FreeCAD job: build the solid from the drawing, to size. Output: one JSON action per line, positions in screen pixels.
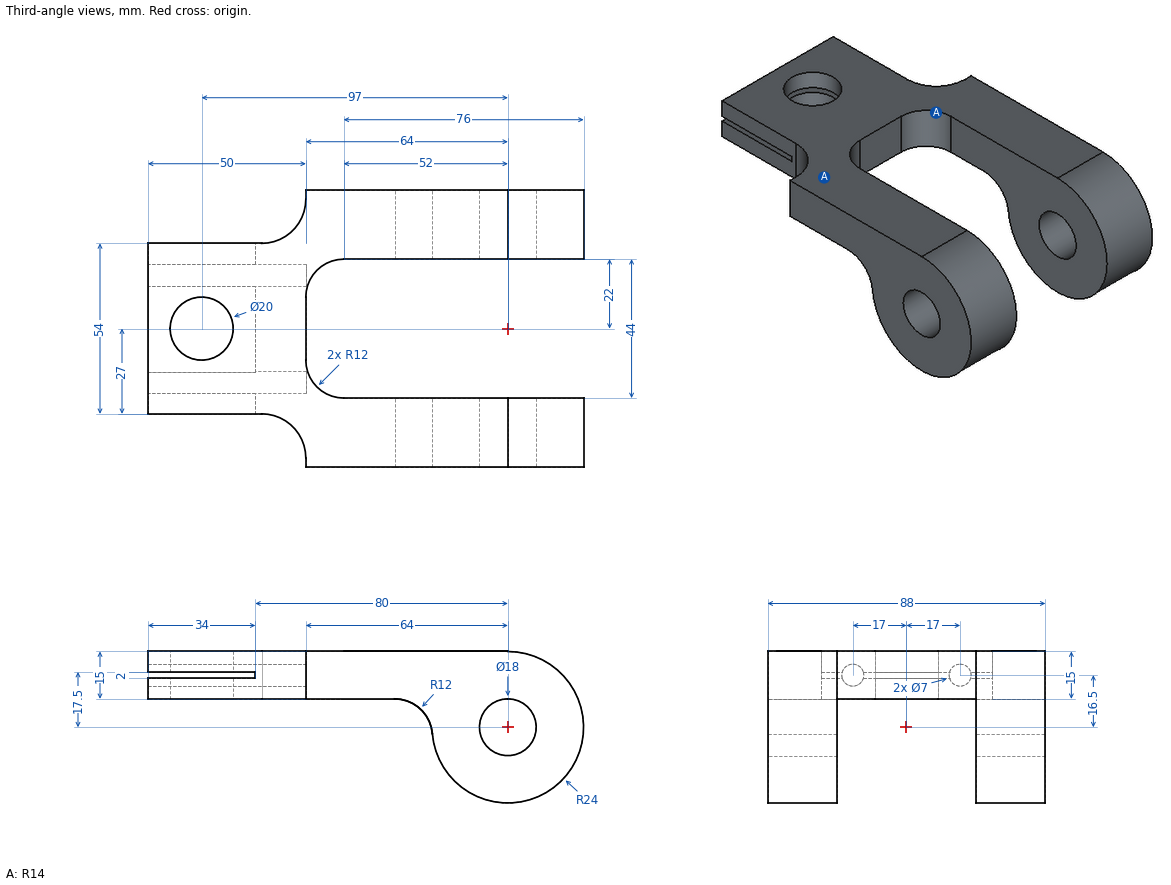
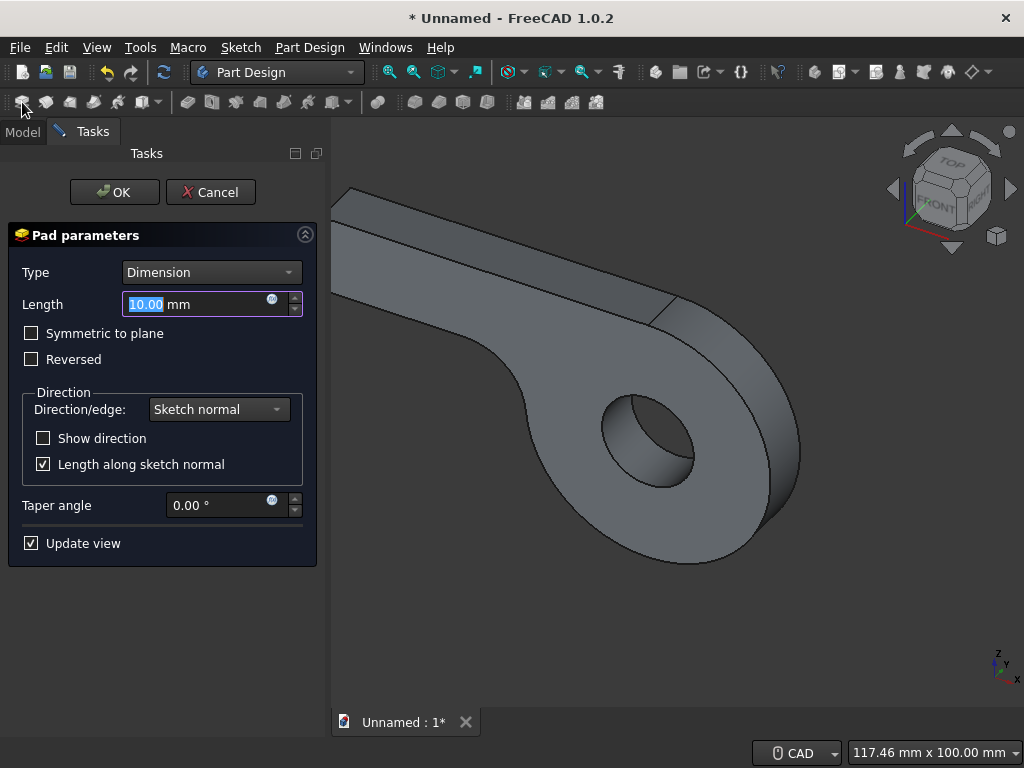
{"action": "type", "text": "88"}
{"action": "key", "text": "Tab"}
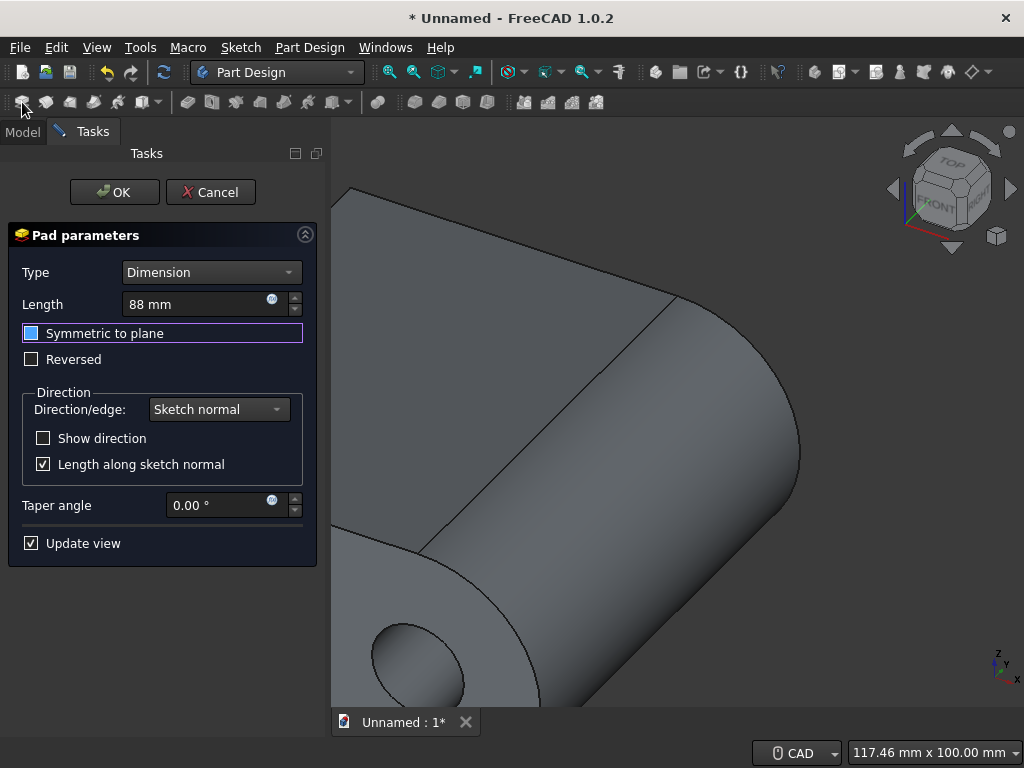
{"action": "left_click", "coordinate": [30, 333]}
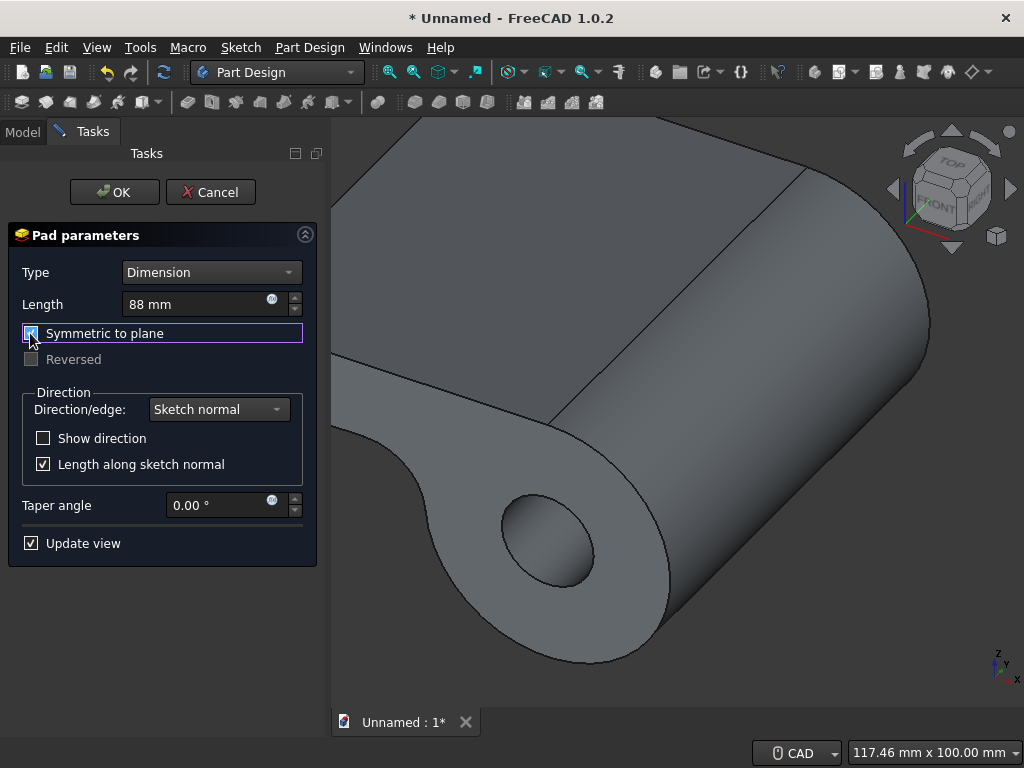
{"action": "left_click", "coordinate": [115, 192]}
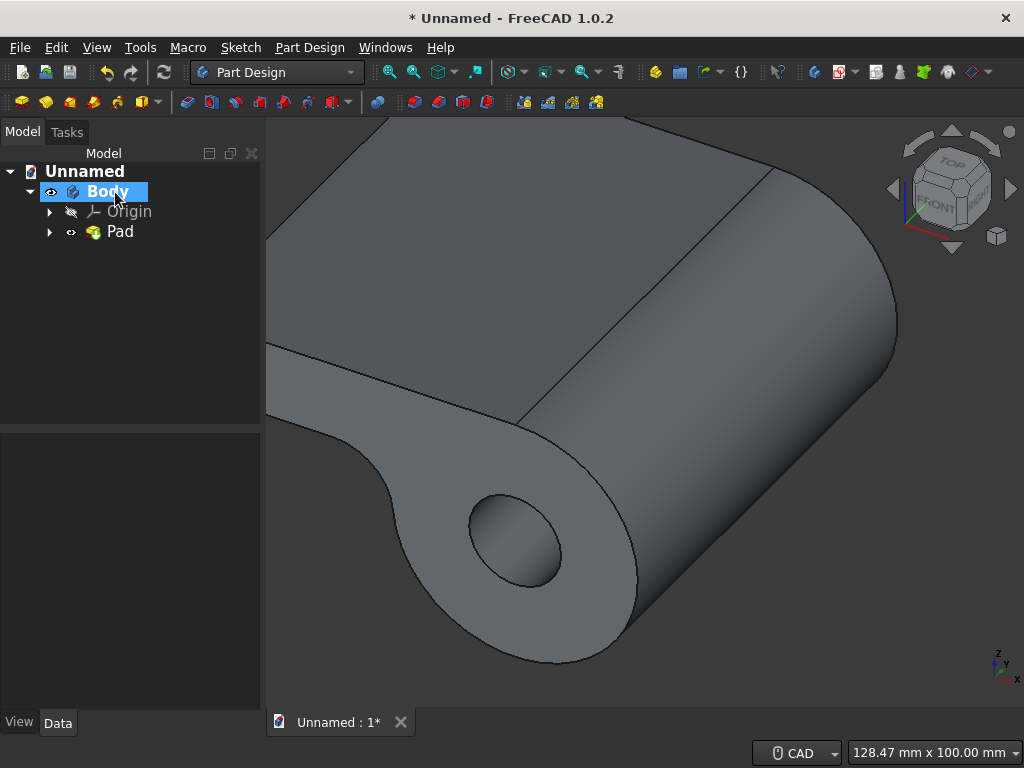
{"action": "left_click", "coordinate": [390, 72]}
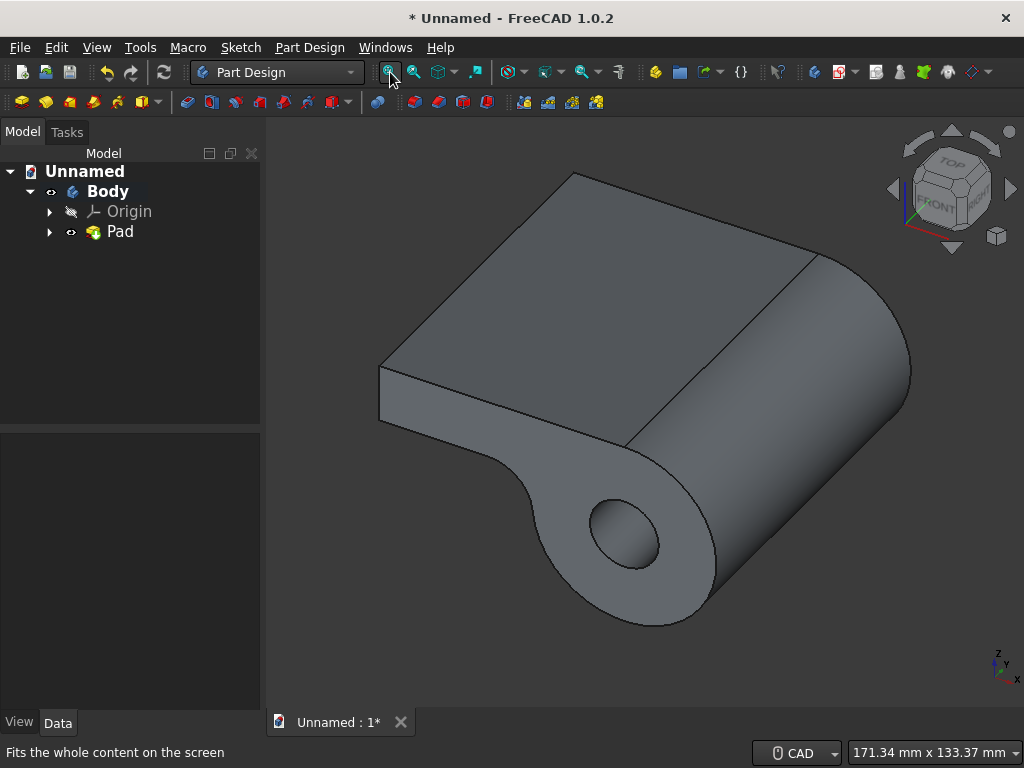
{"action": "key", "text": "5"}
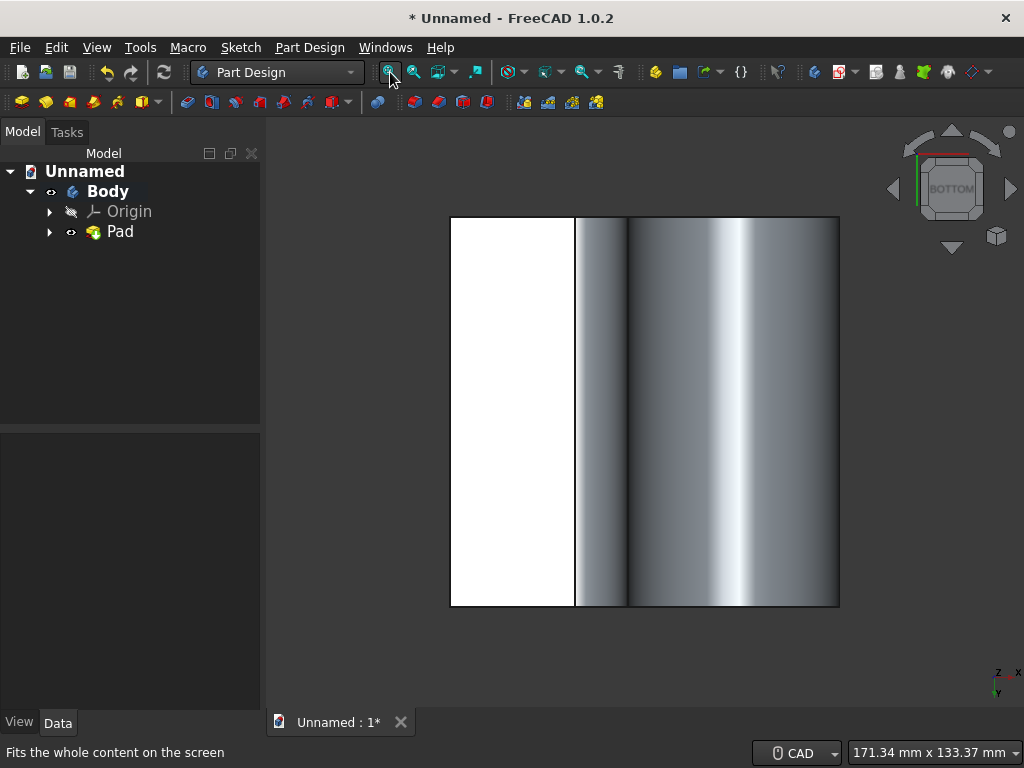
{"action": "left_click", "coordinate": [513, 522]}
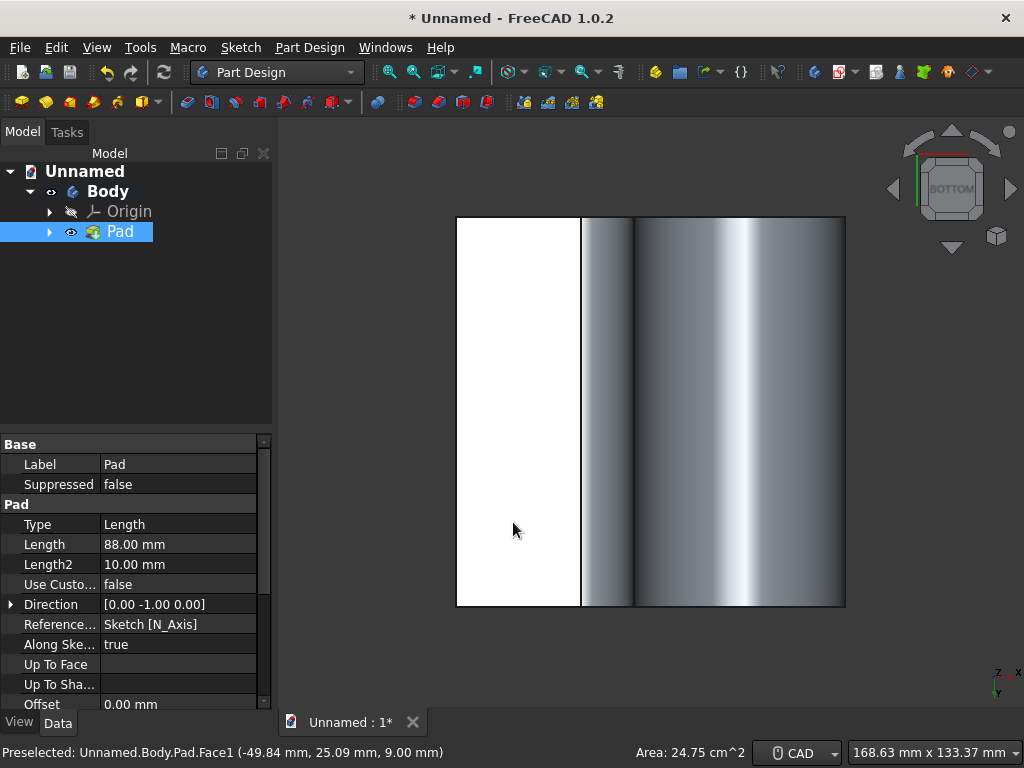
{"action": "left_click", "coordinate": [840, 72]}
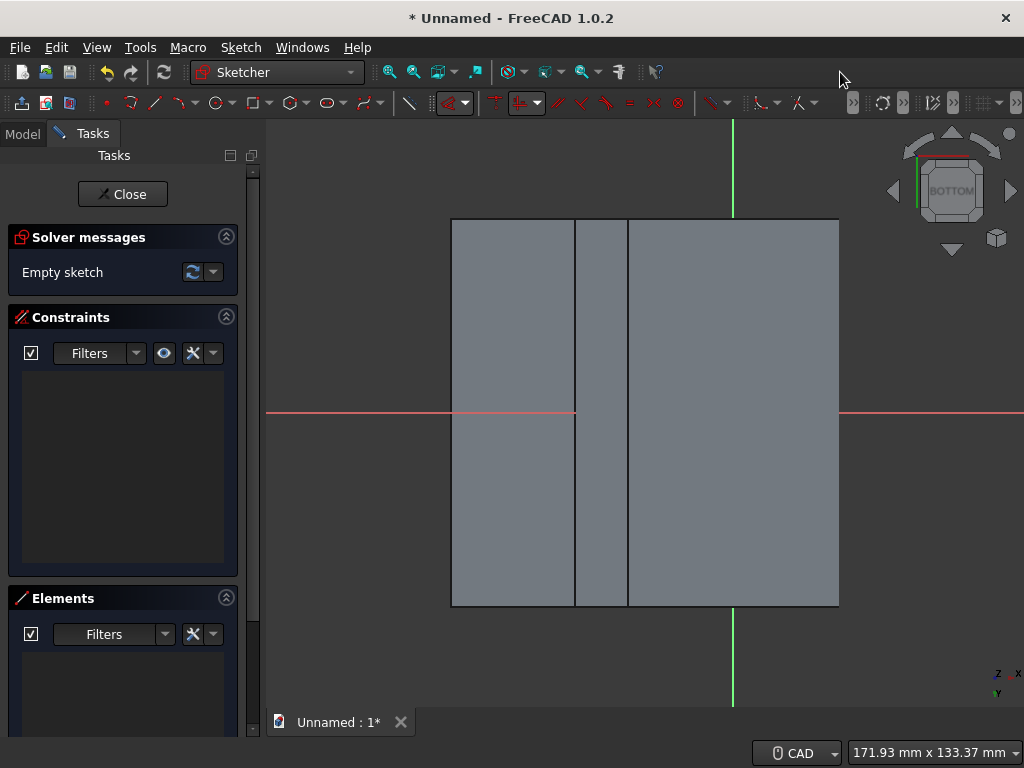
{"action": "scroll", "coordinate": [859, 413], "scroll_direction": "down", "scroll_amount": 1}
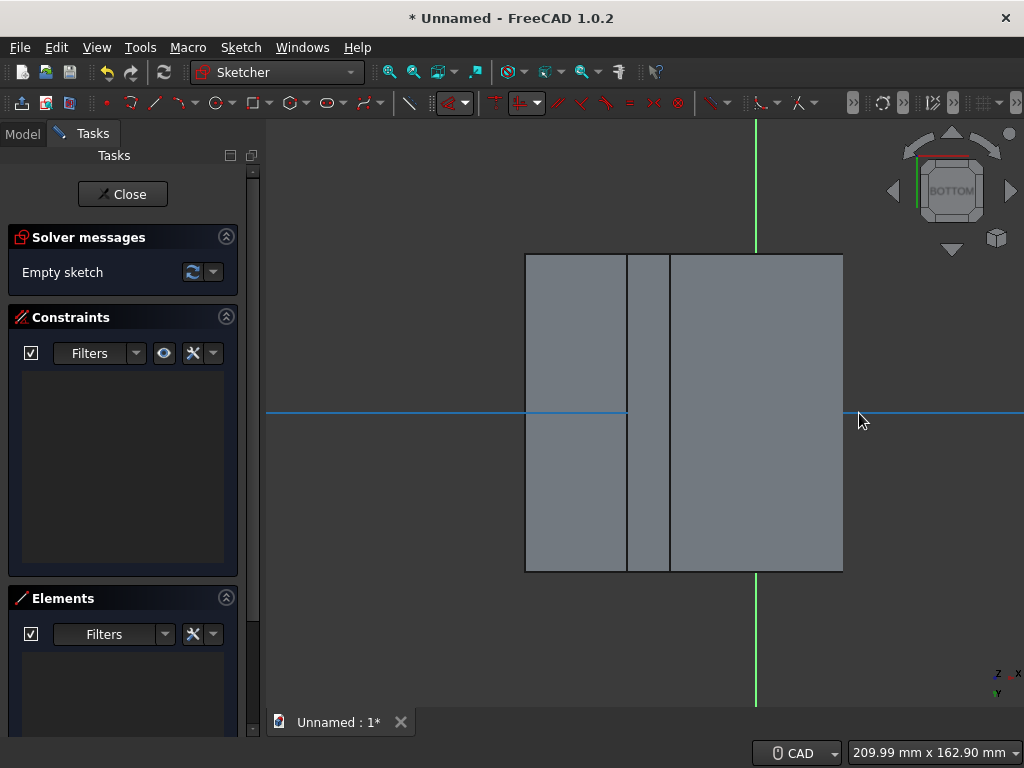
{"action": "left_click", "coordinate": [254, 104]}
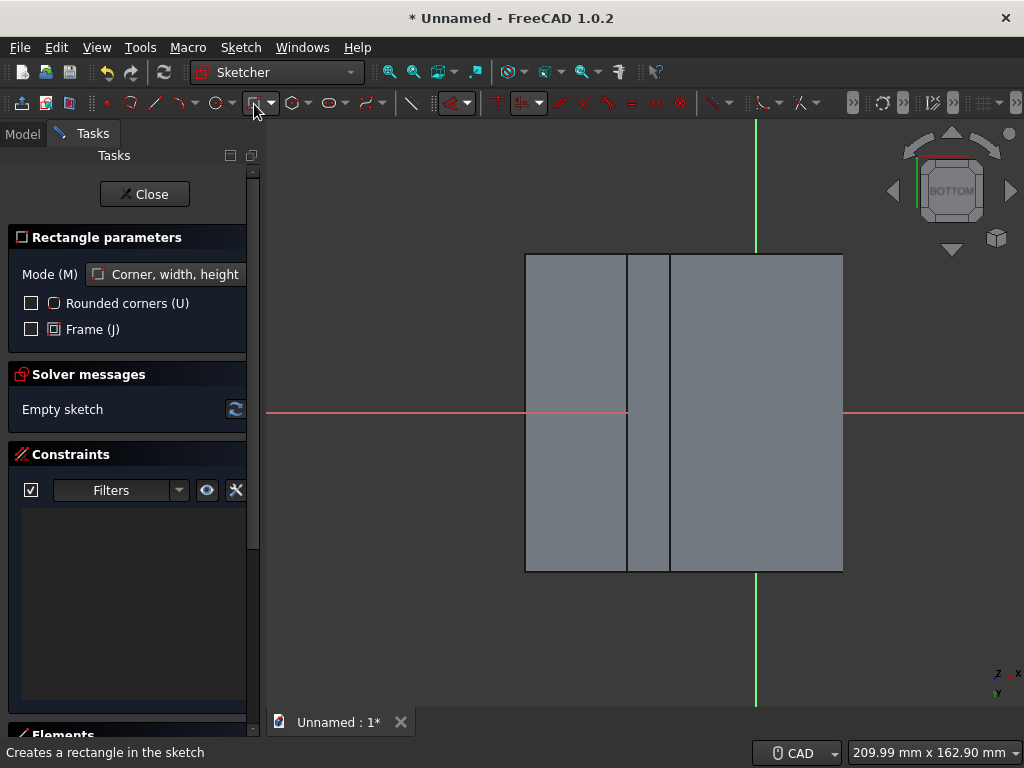
{"action": "left_click", "coordinate": [345, 316]}
{"action": "left_click", "coordinate": [525, 511]}
{"action": "key", "text": "Escape"}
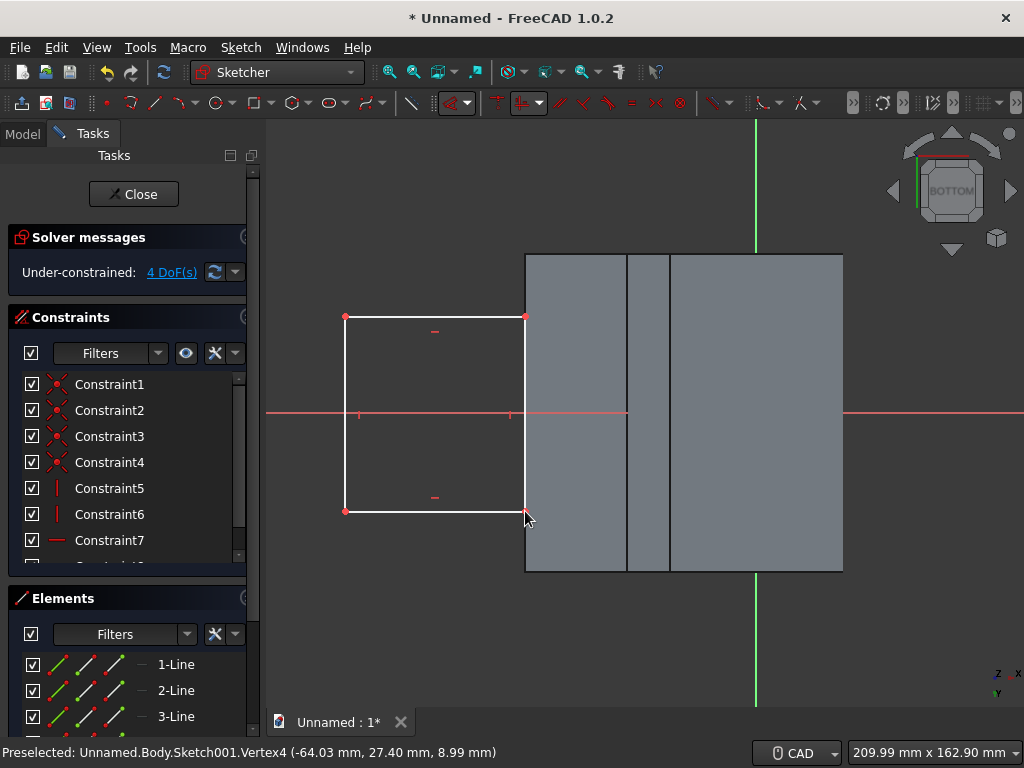
{"action": "left_click", "coordinate": [345, 376]}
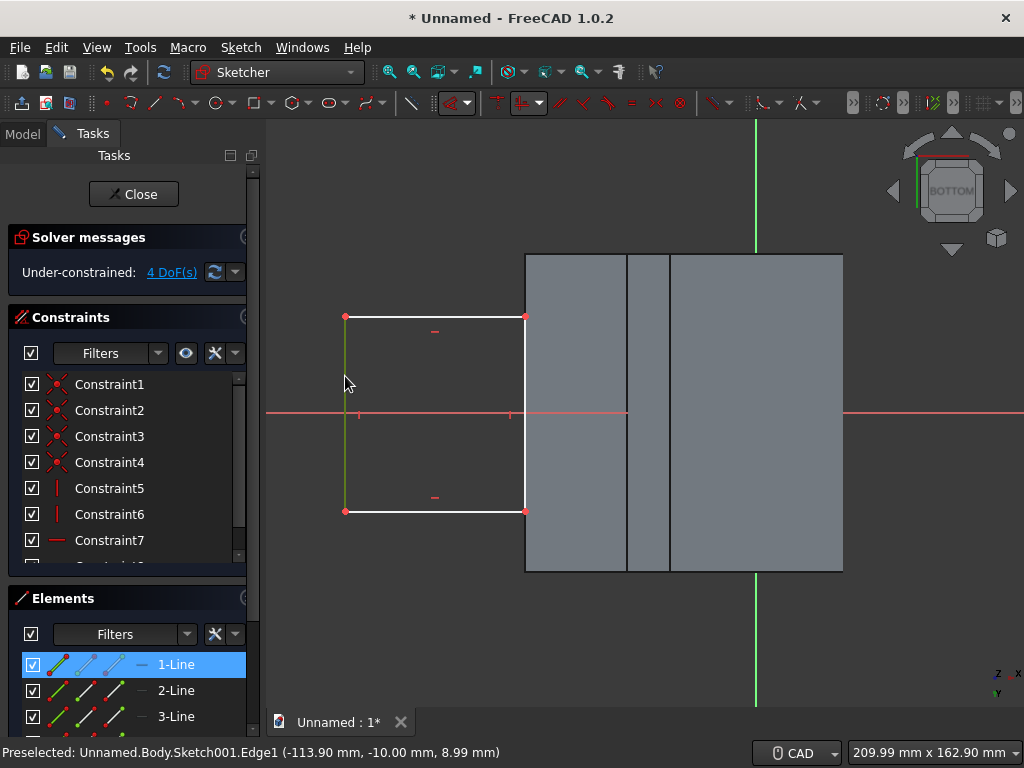
{"action": "key", "text": "i"}